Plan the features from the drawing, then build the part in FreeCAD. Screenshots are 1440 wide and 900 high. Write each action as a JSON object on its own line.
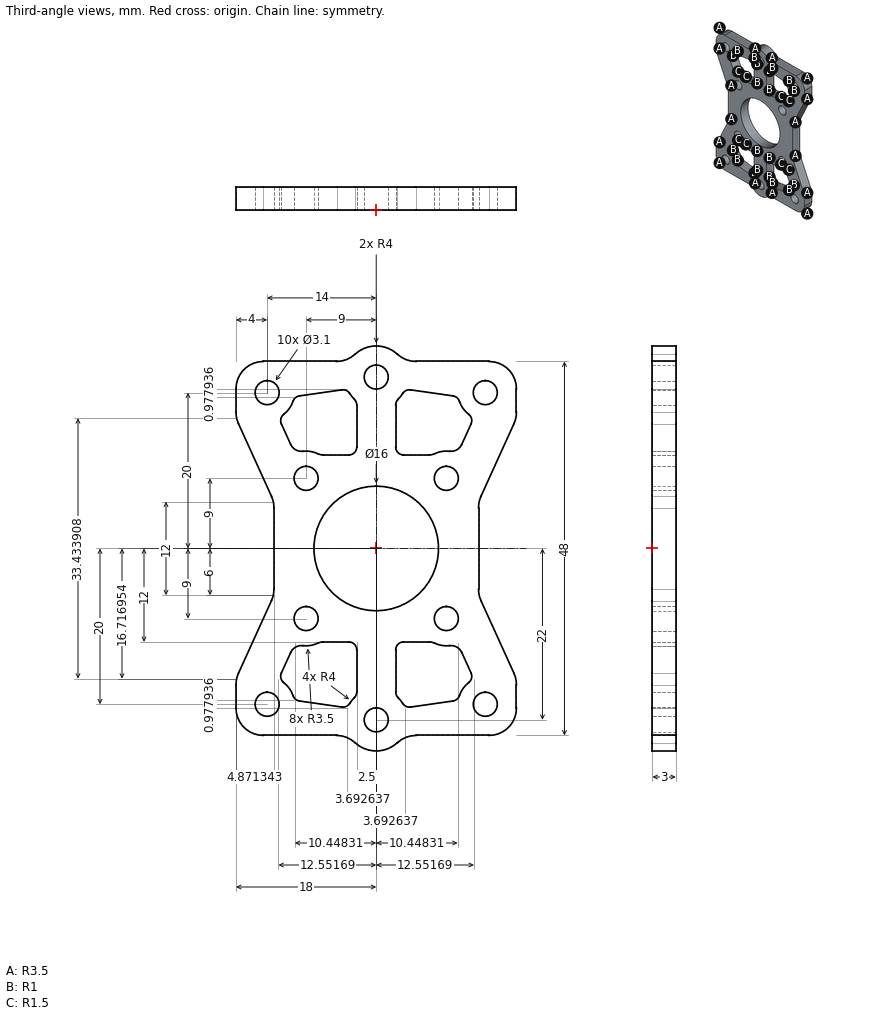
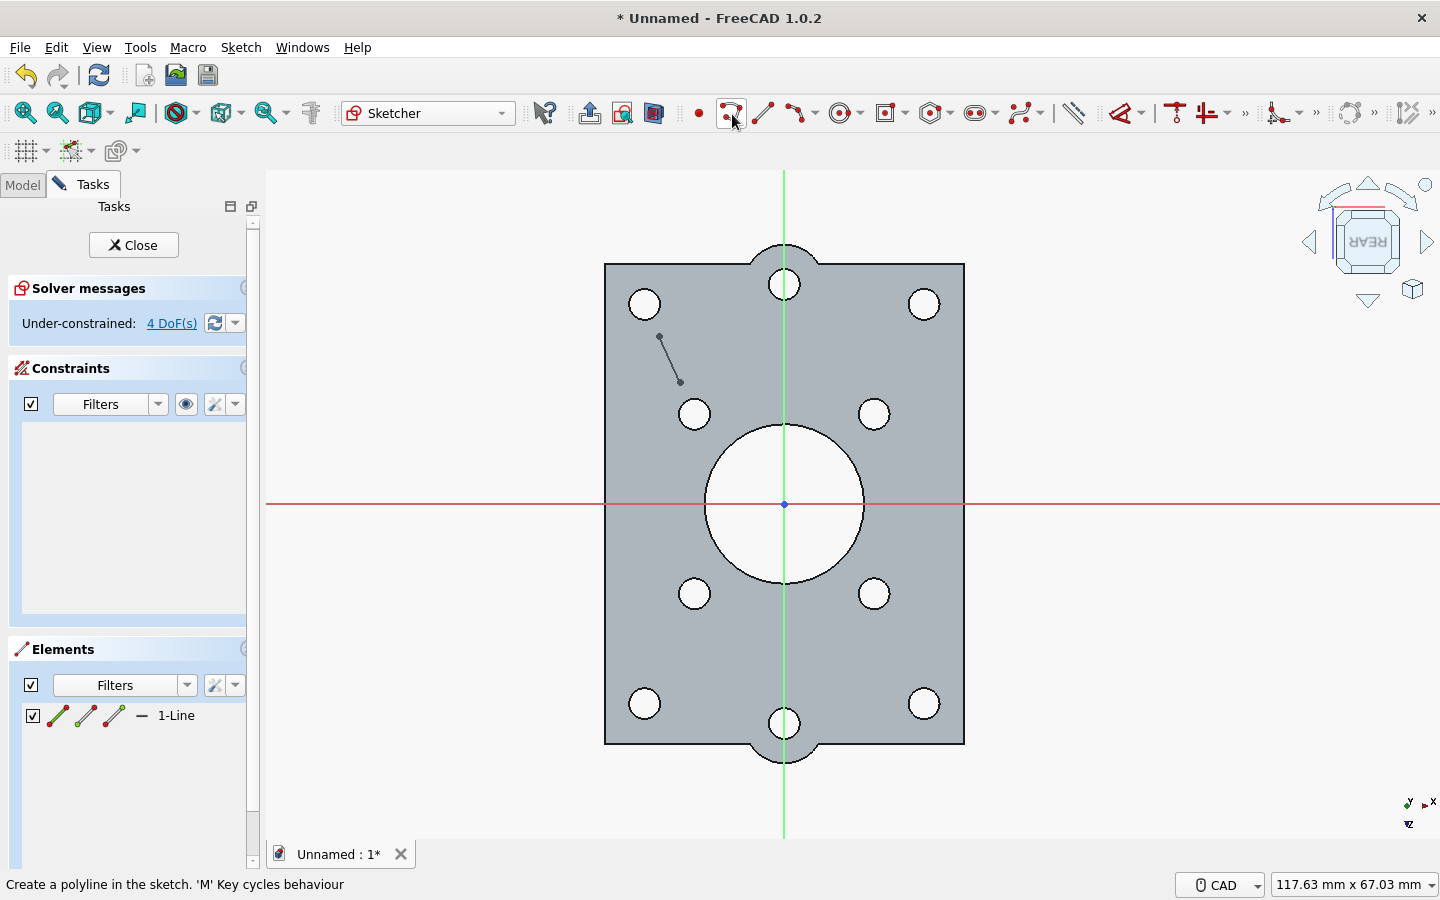
{"action": "left_click", "coordinate": [713, 384]}
{"action": "left_click", "coordinate": [759, 384]}
{"action": "left_click", "coordinate": [759, 316]}
{"action": "right_click", "coordinate": [759, 316]}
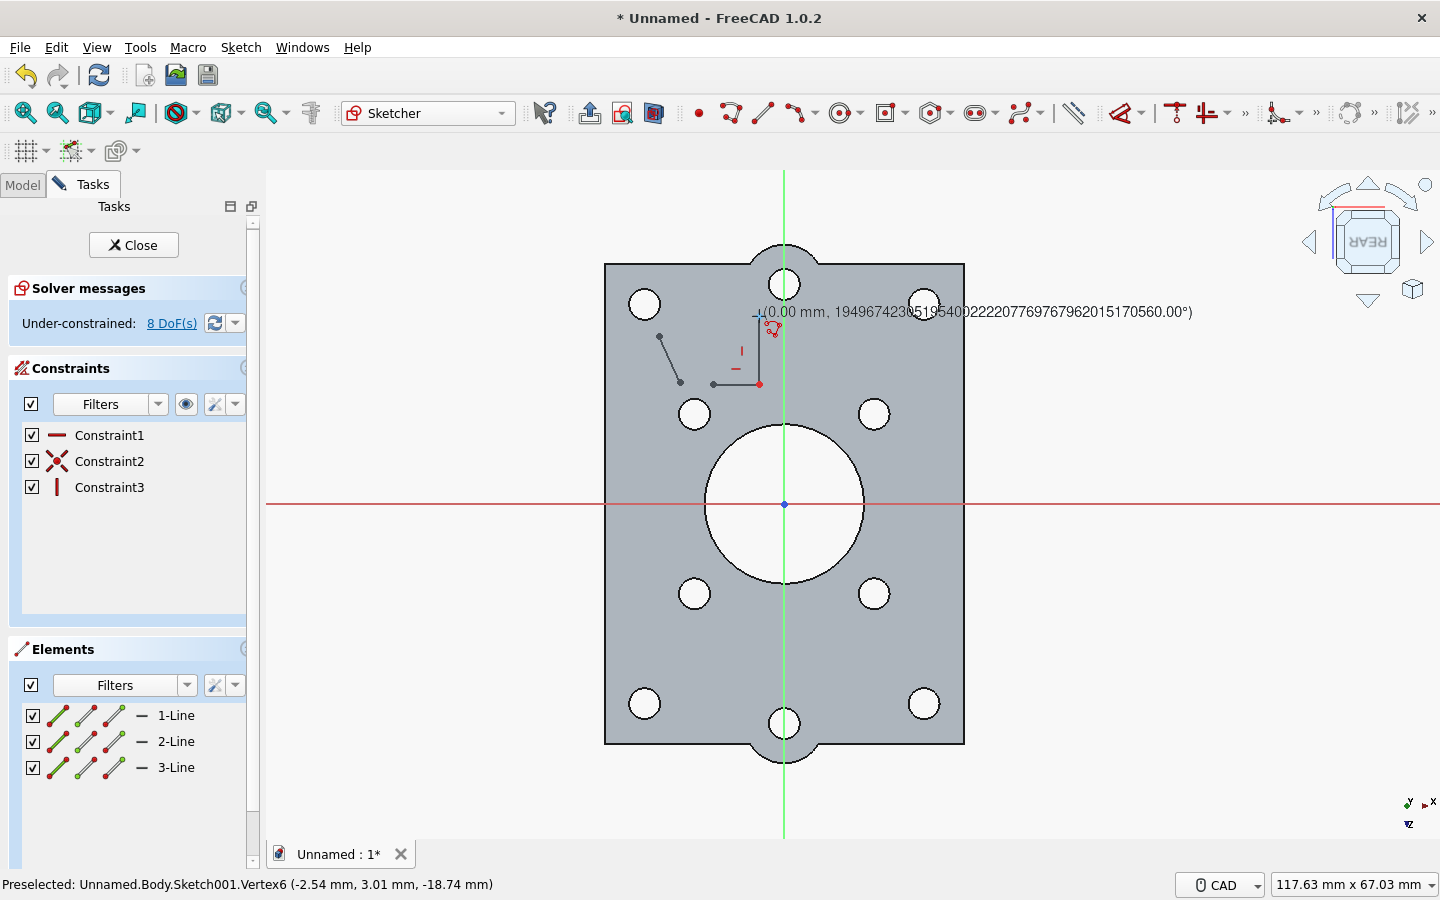
{"action": "key", "text": "g l"}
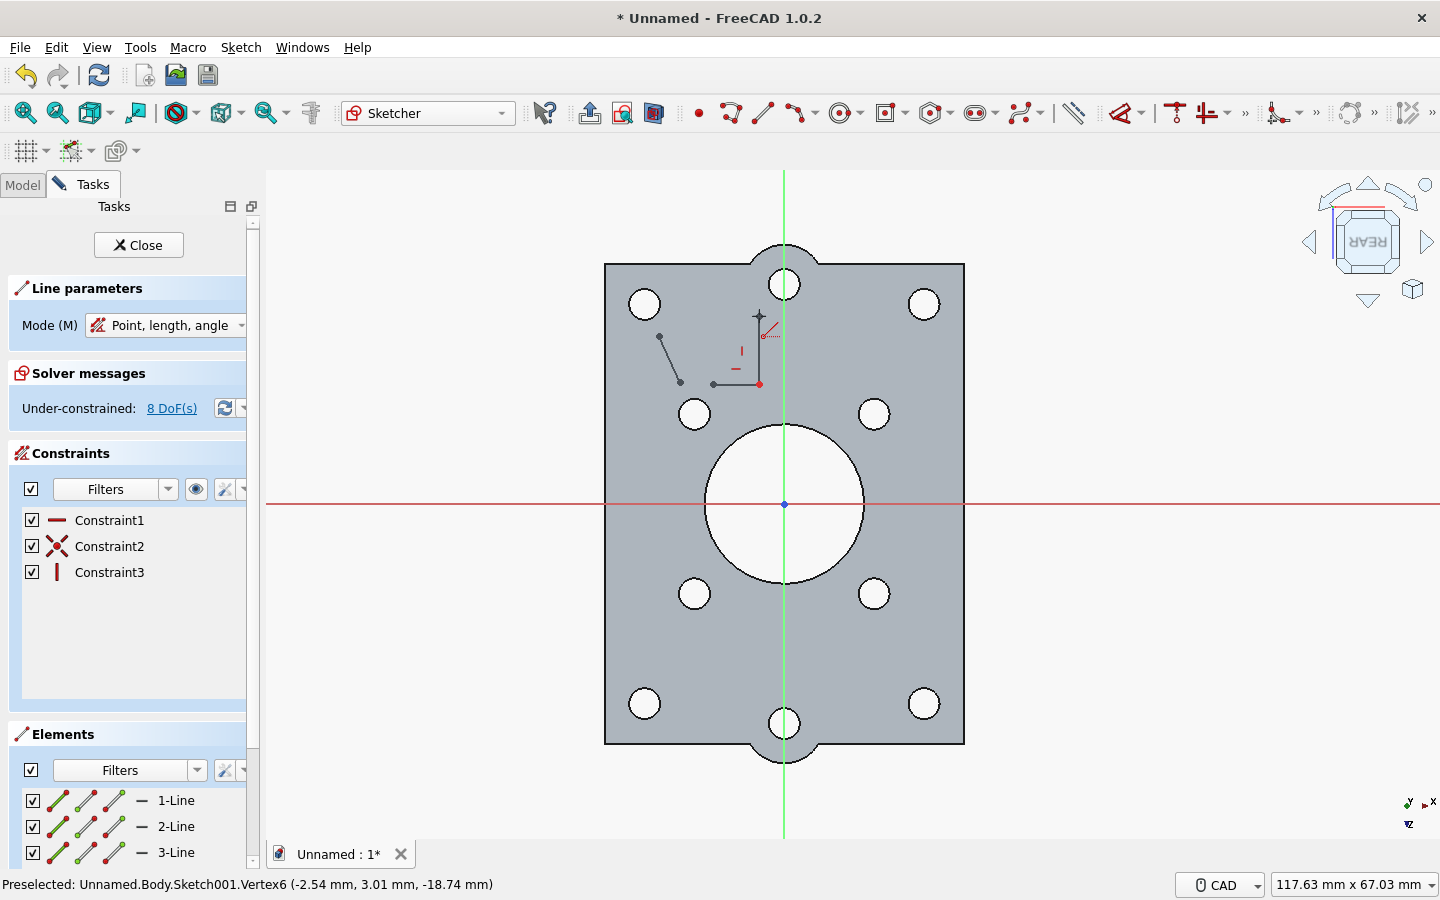
{"action": "left_click", "coordinate": [747, 300]}
{"action": "left_click", "coordinate": [679, 310]}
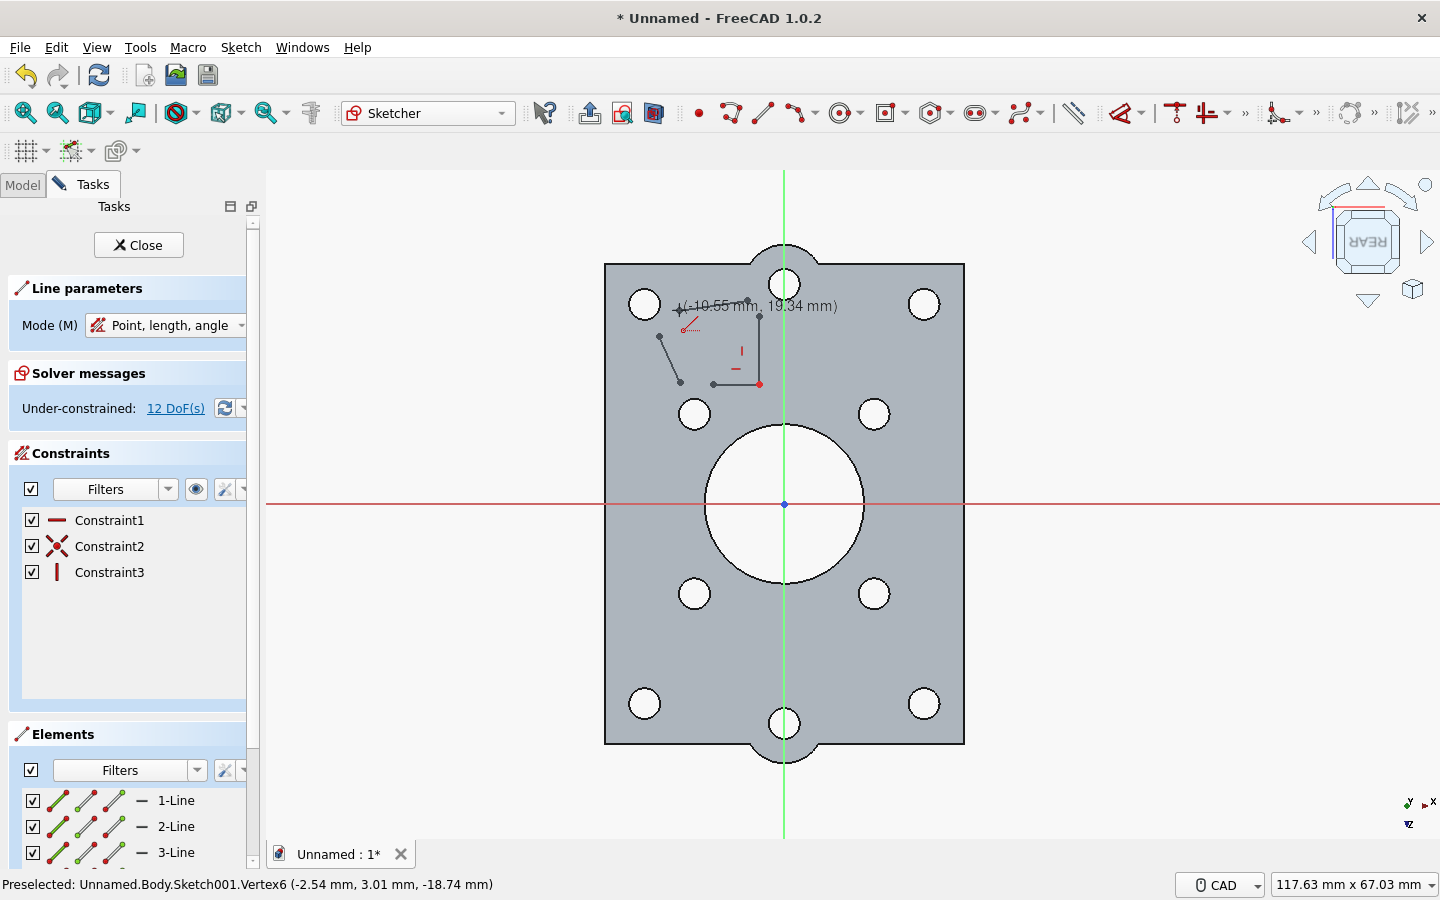
{"action": "left_click", "coordinate": [796, 114]}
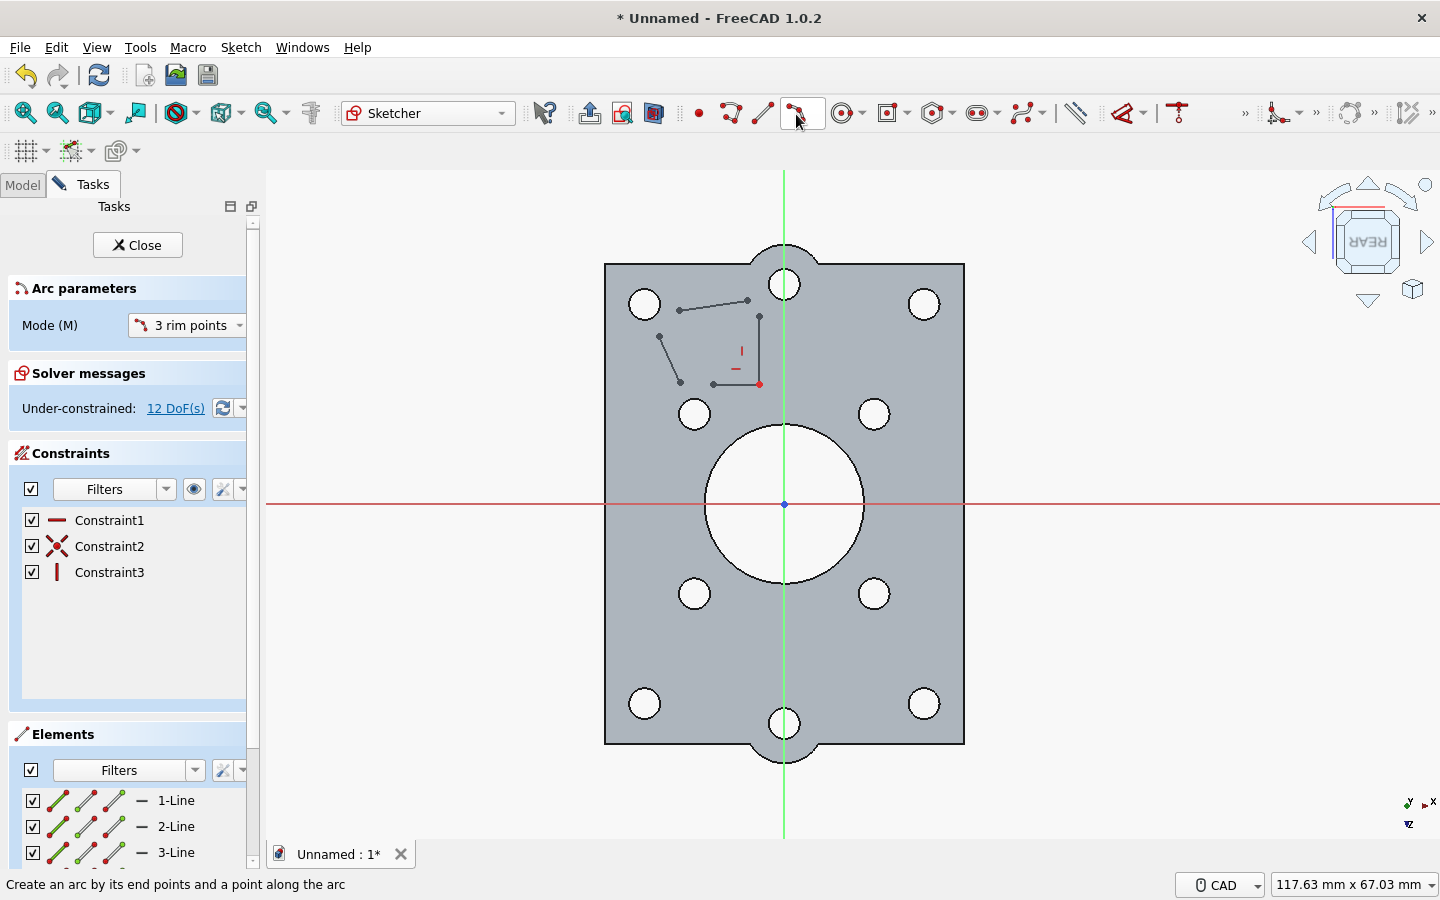
{"action": "left_click", "coordinate": [680, 383]}
{"action": "left_click", "coordinate": [713, 385]}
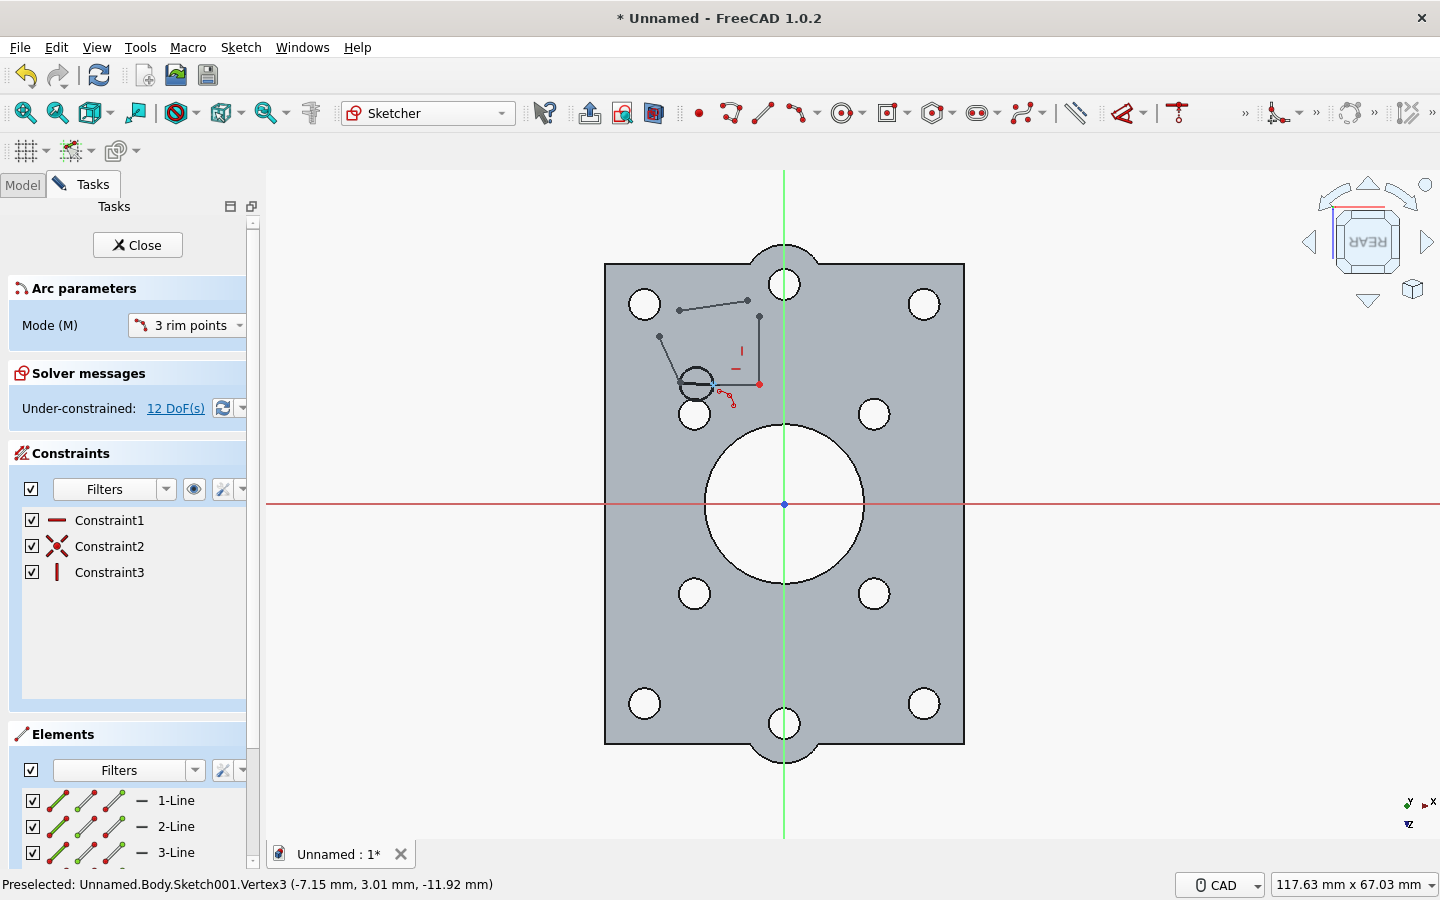
{"action": "scroll", "coordinate": [697, 379], "scroll_direction": "up", "scroll_amount": 7}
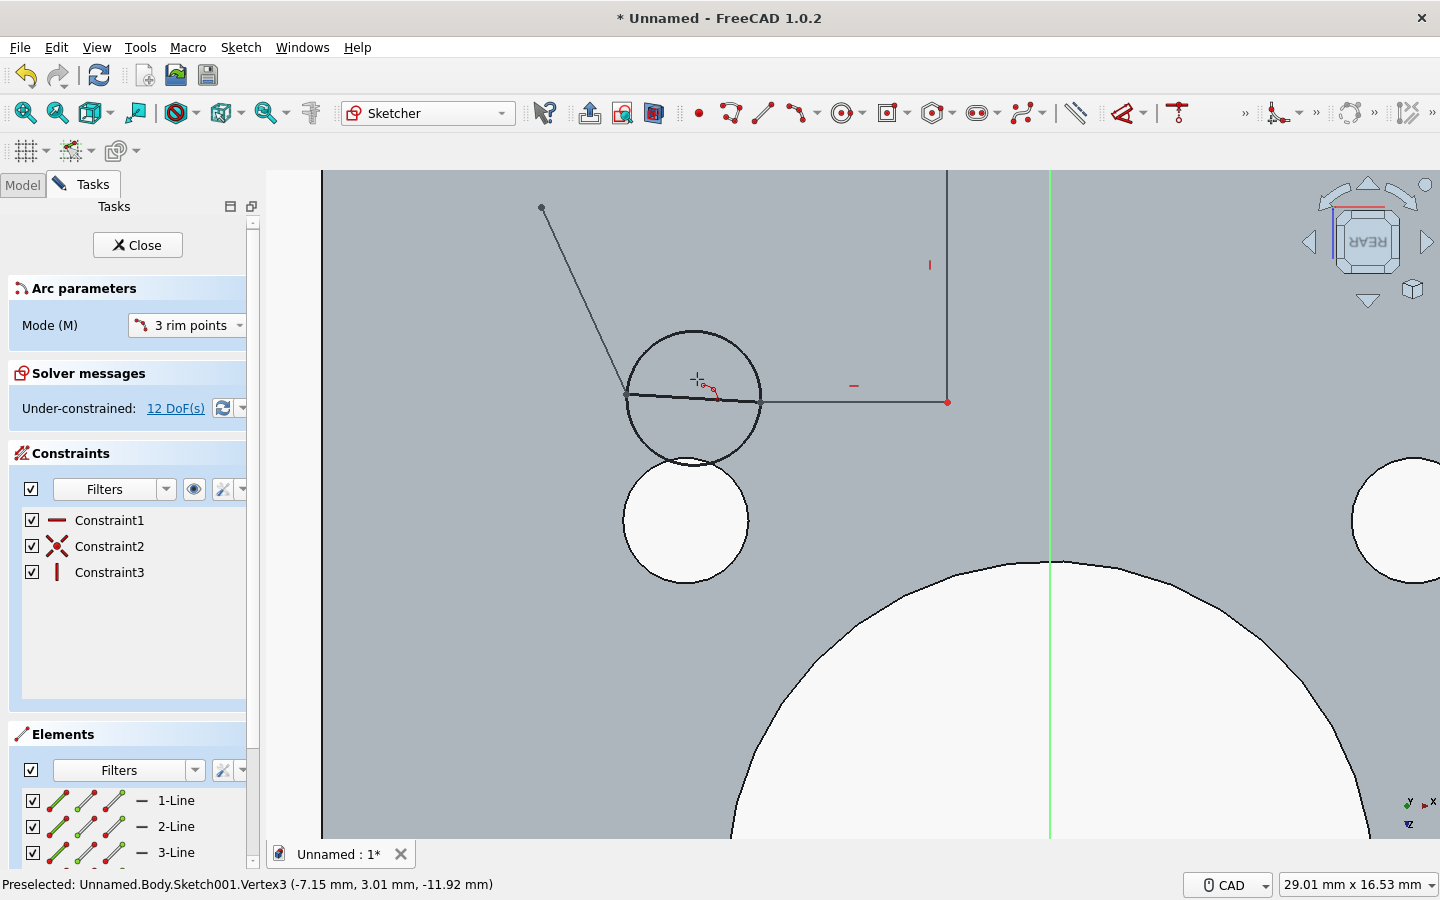
{"action": "left_click", "coordinate": [694, 379]}